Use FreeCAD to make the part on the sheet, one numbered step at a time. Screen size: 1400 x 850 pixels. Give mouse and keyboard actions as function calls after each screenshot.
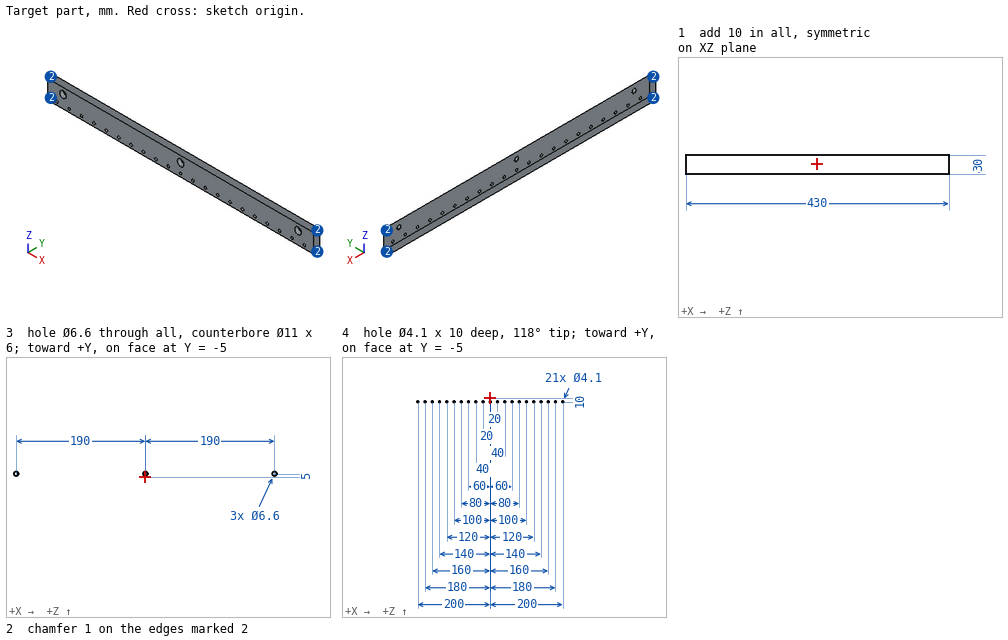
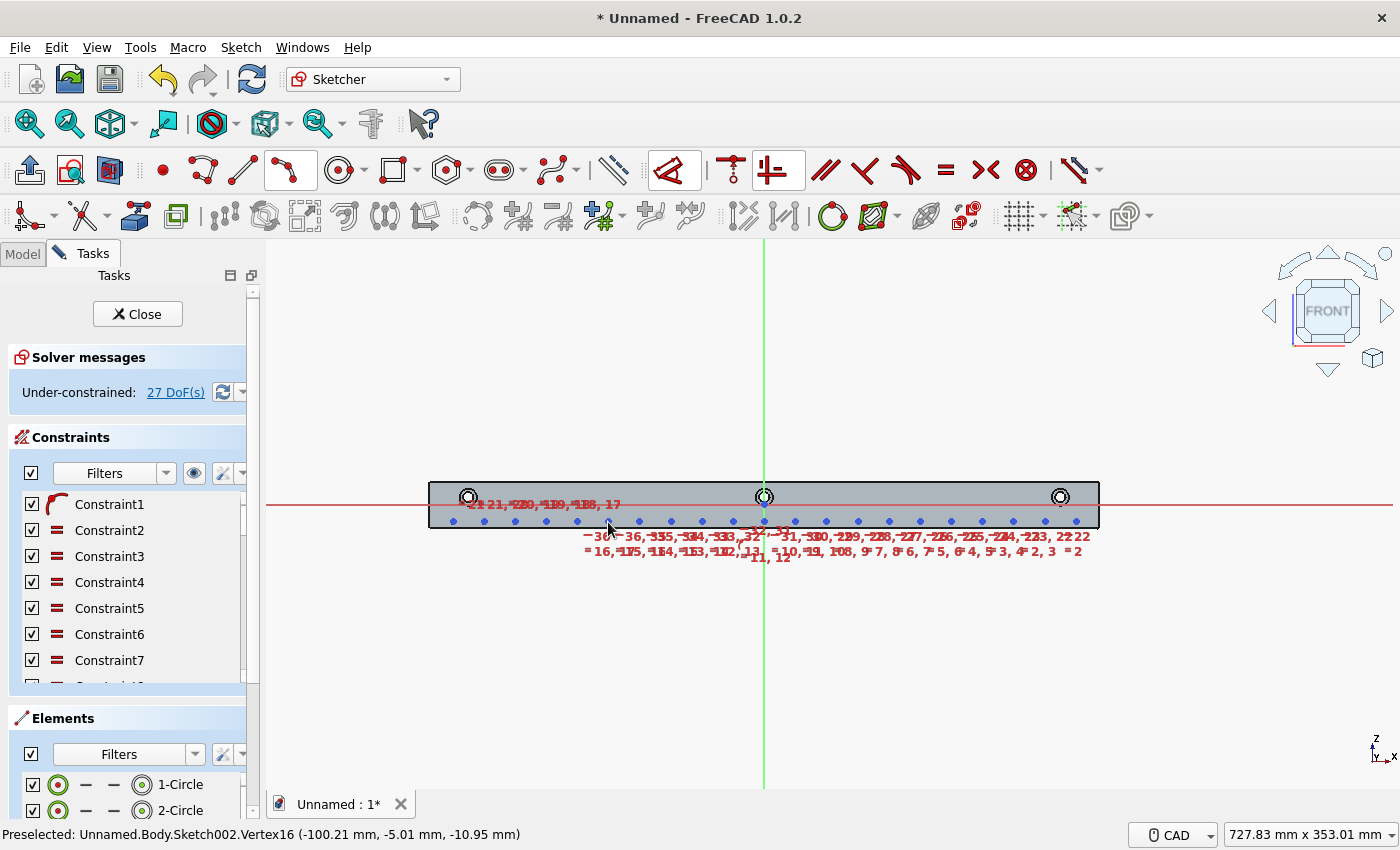
click(608, 522)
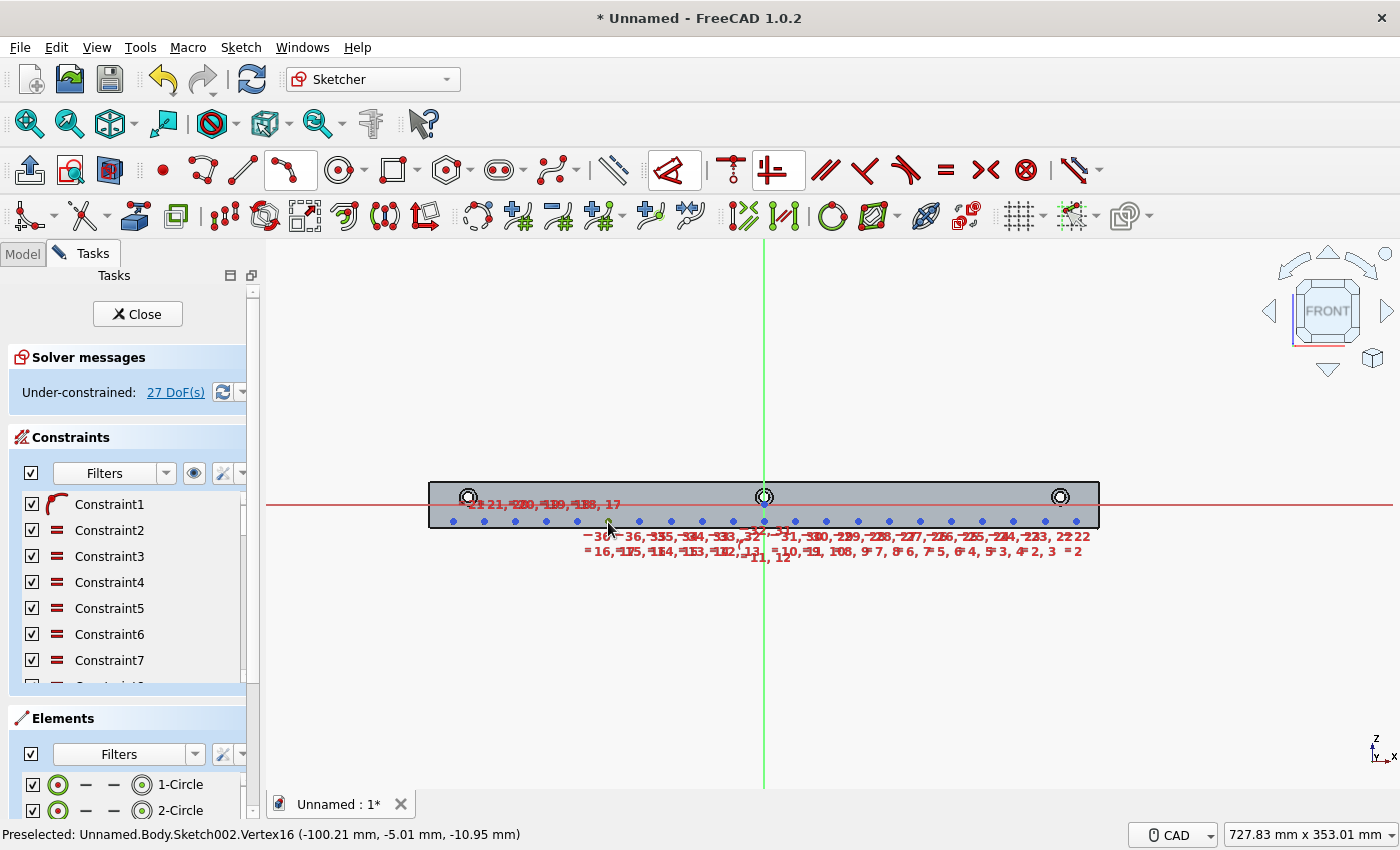
click(577, 522)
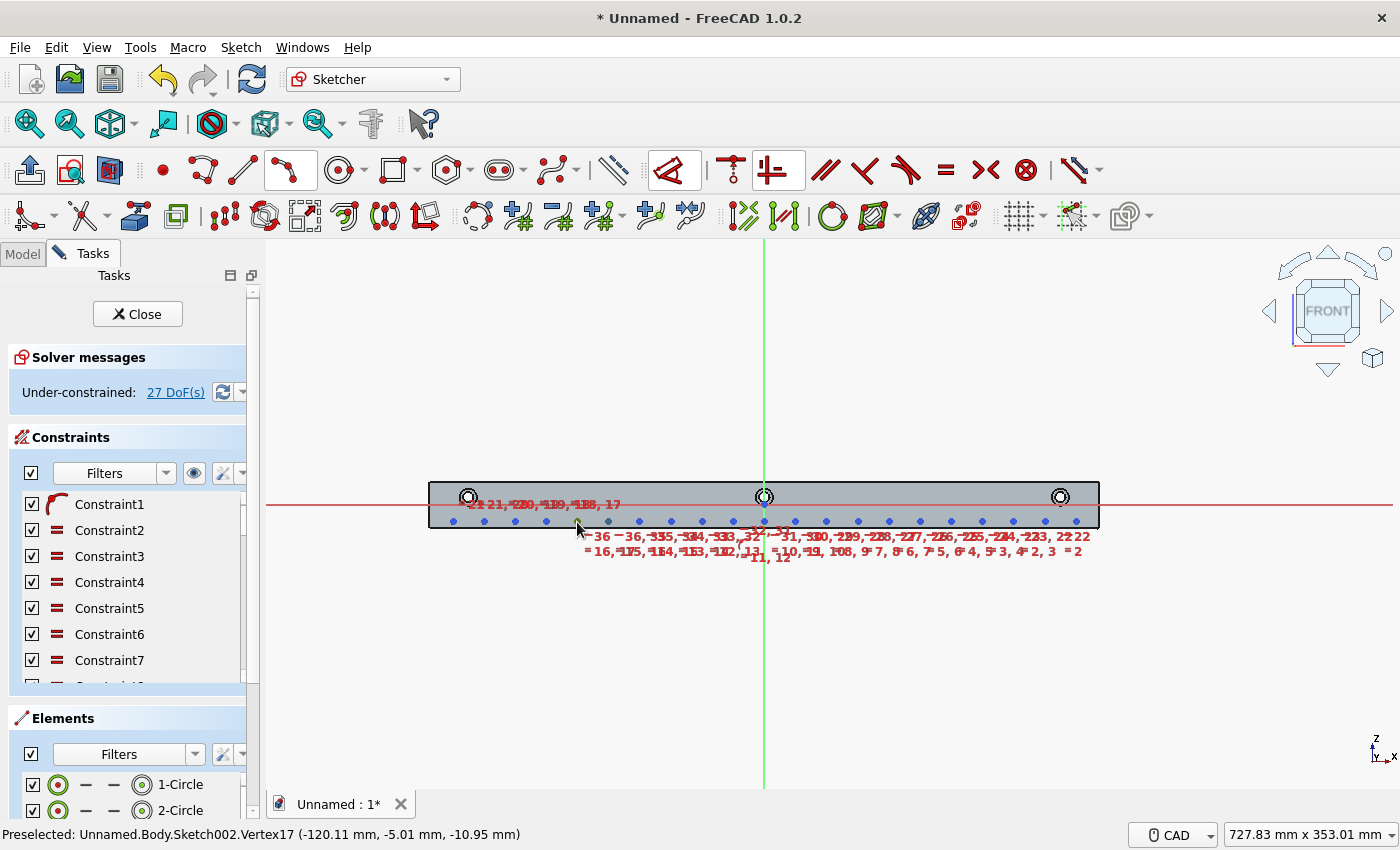
click(800, 170)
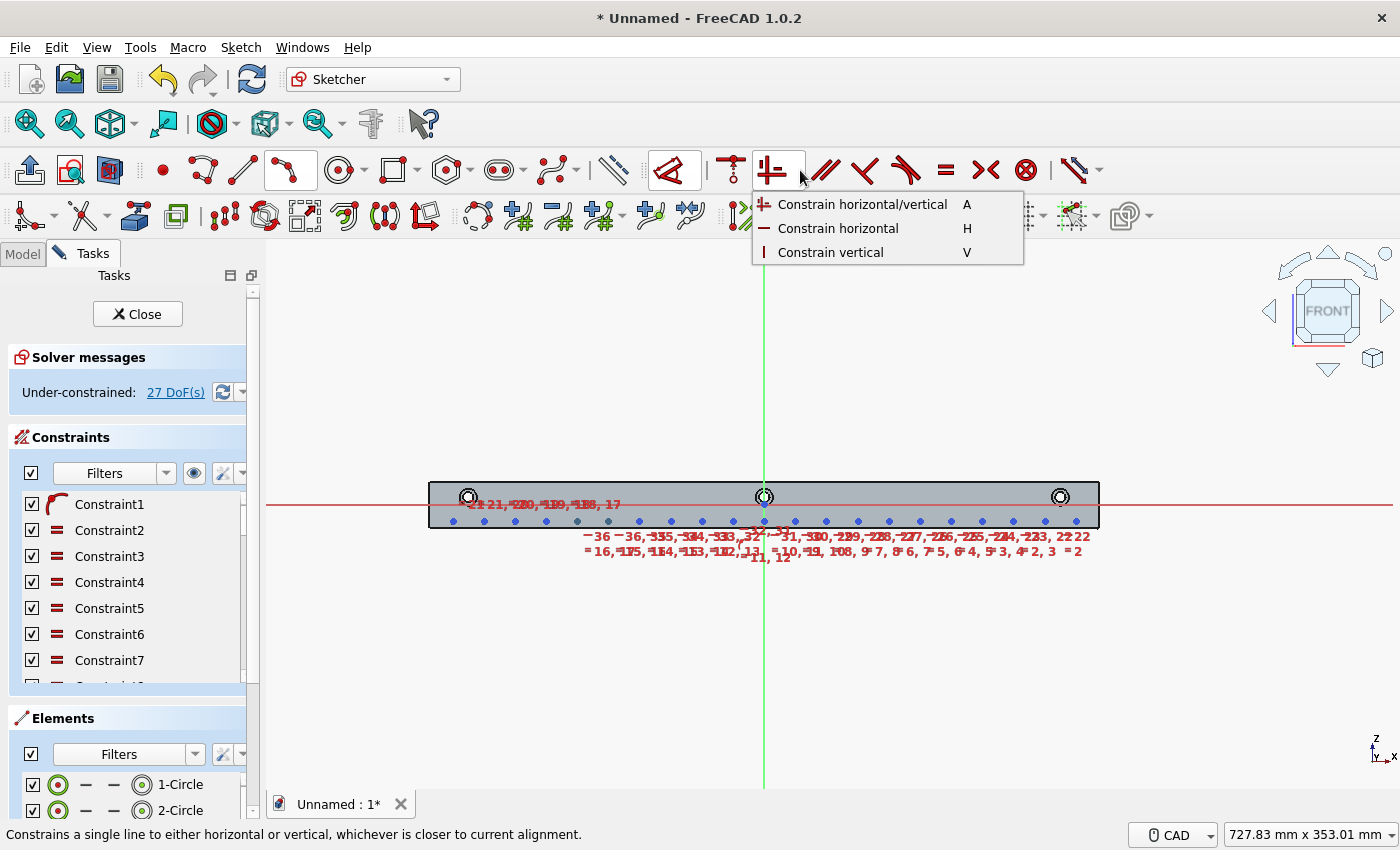
click(888, 228)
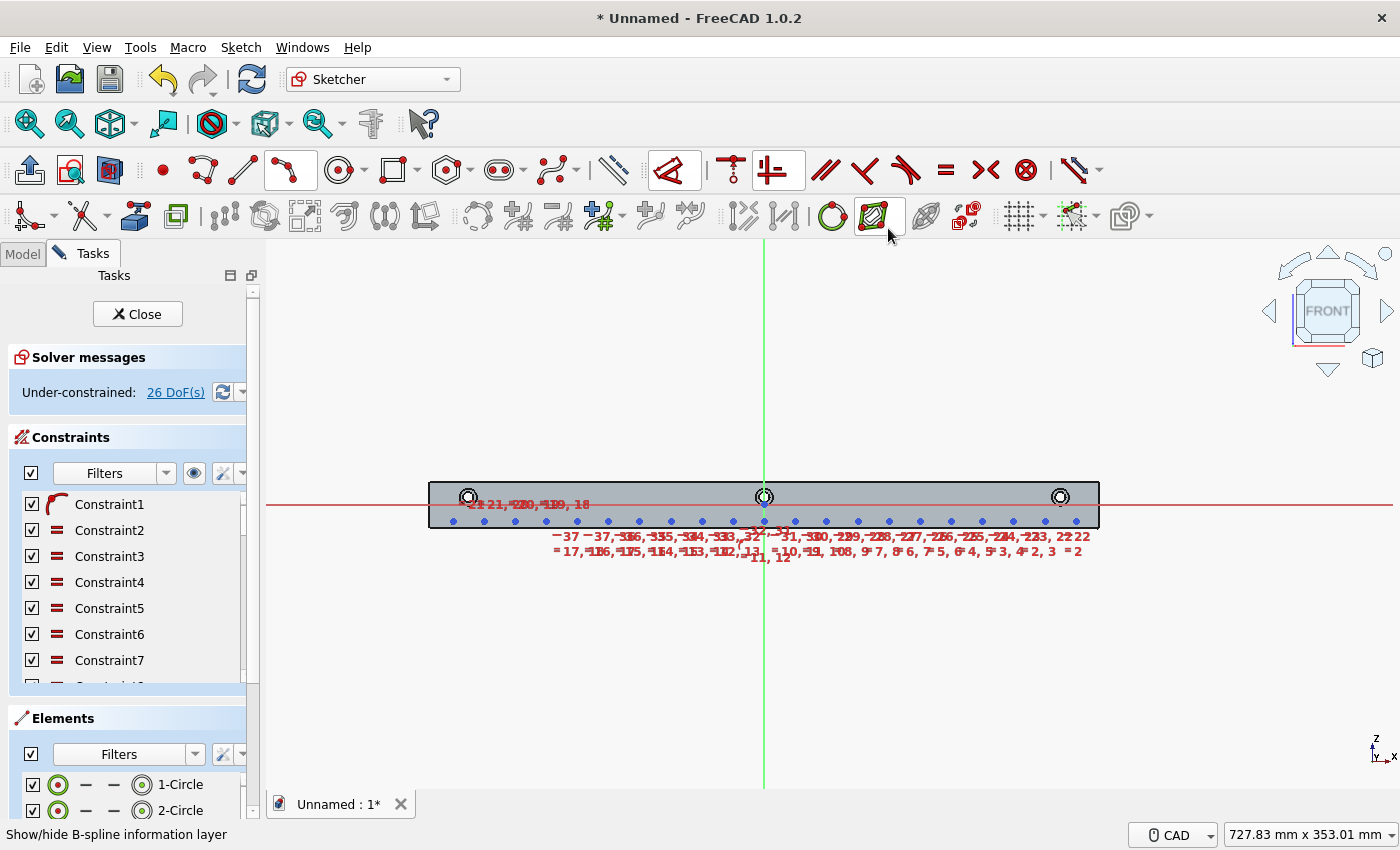
click(577, 522)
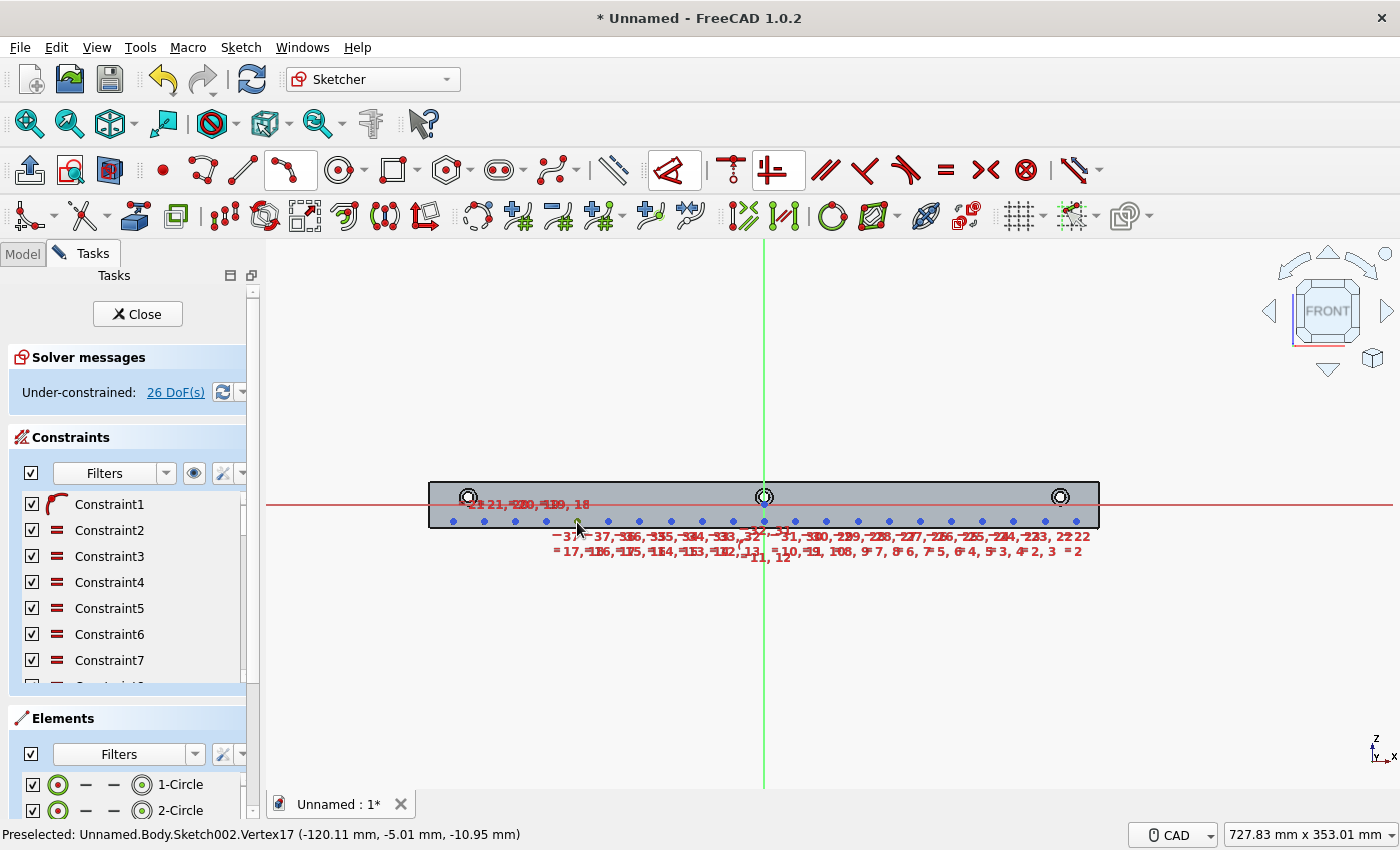
click(546, 522)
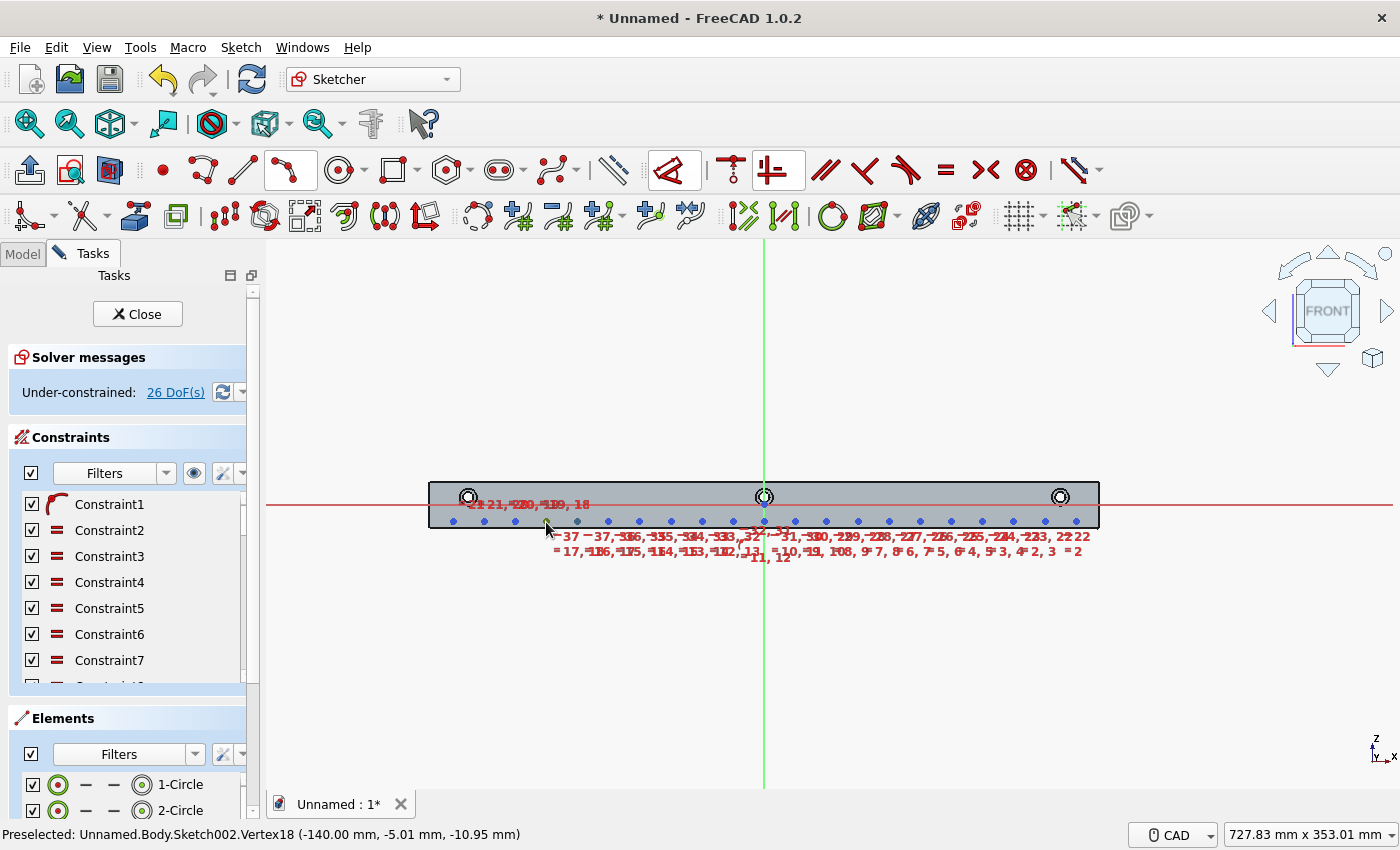
key(h)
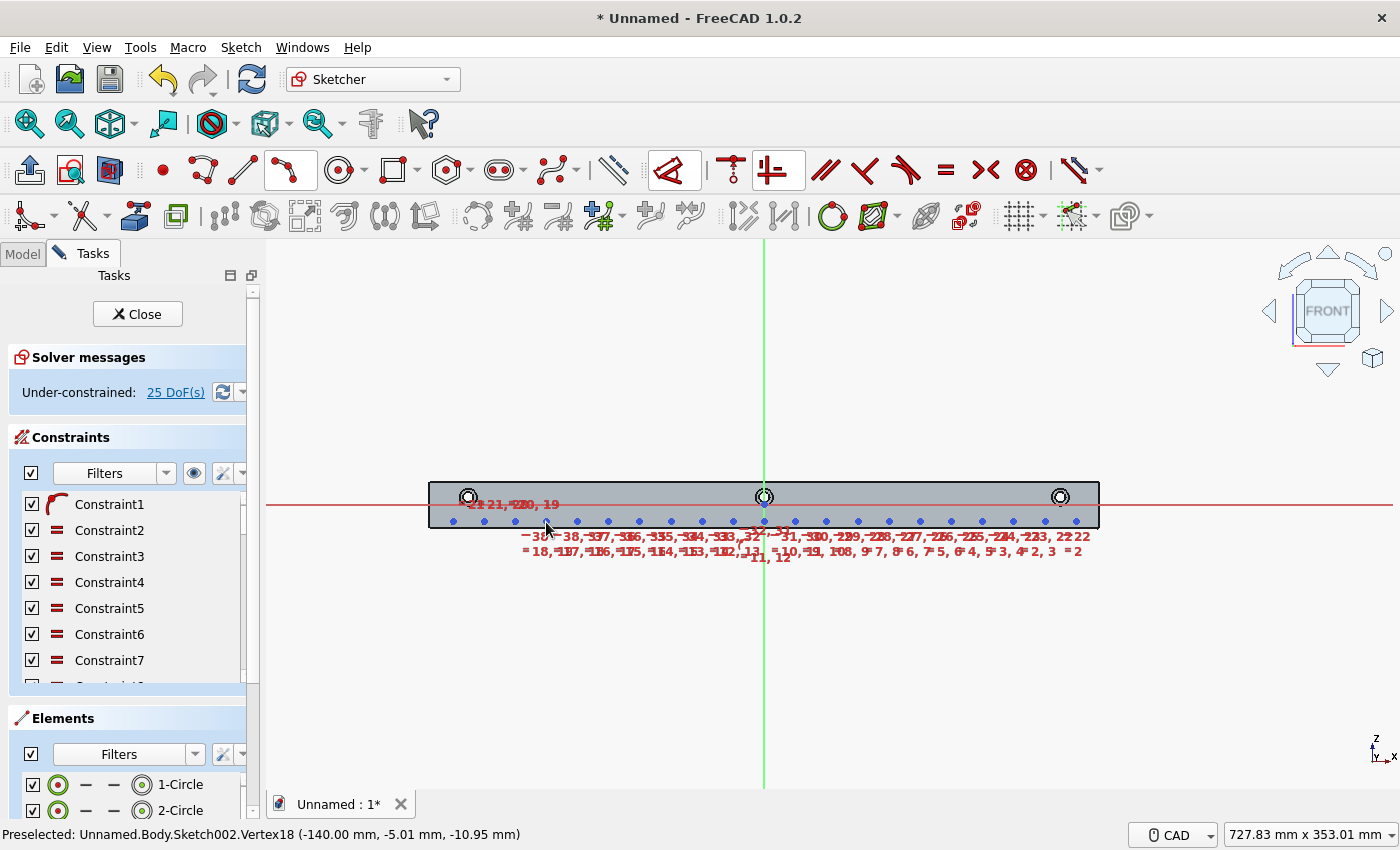
click(546, 522)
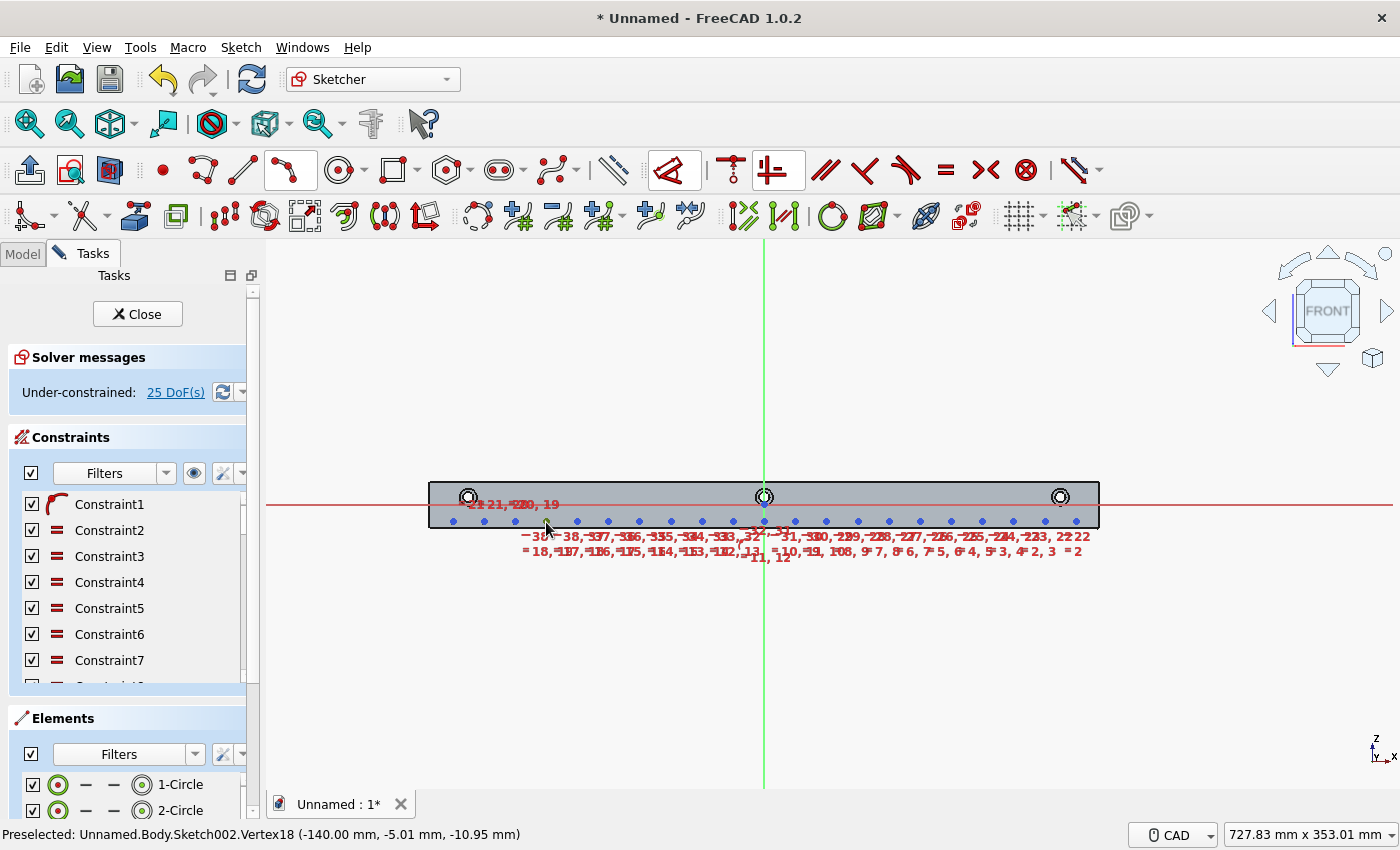
click(515, 522)